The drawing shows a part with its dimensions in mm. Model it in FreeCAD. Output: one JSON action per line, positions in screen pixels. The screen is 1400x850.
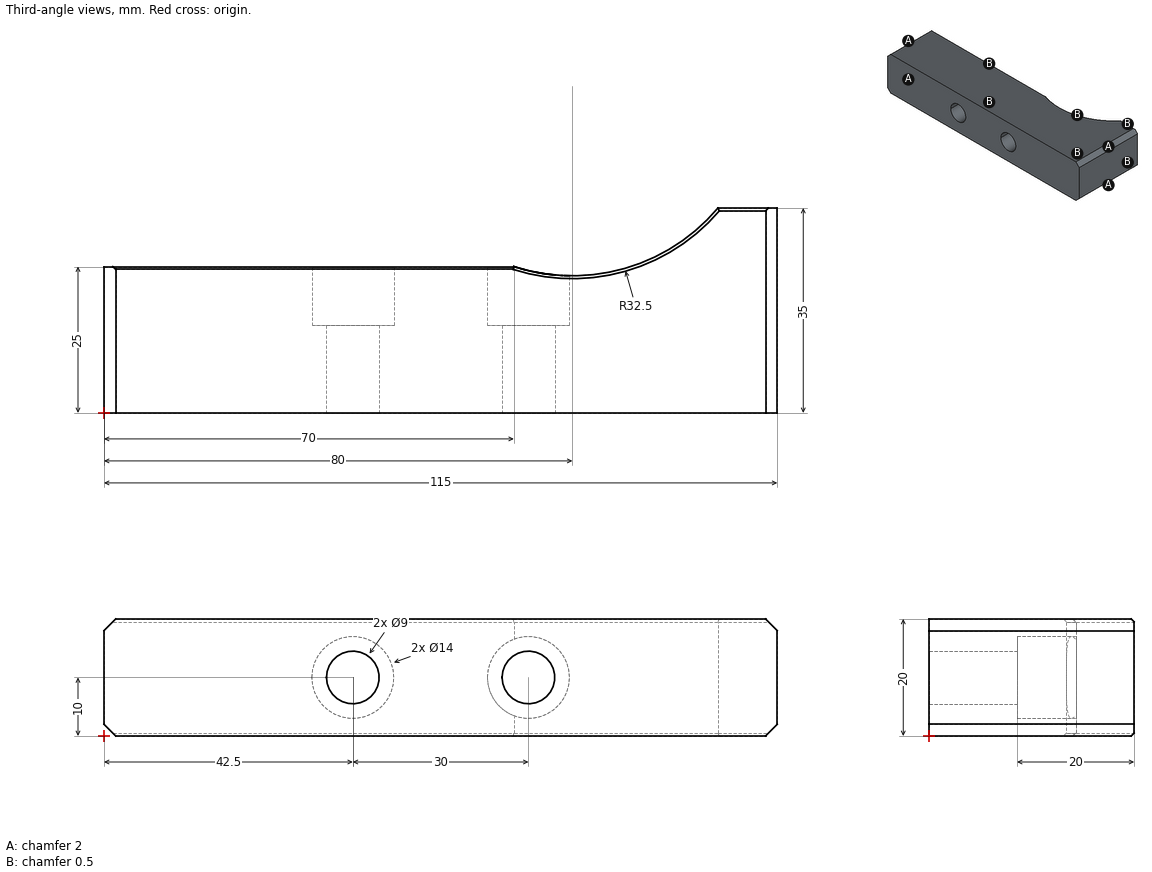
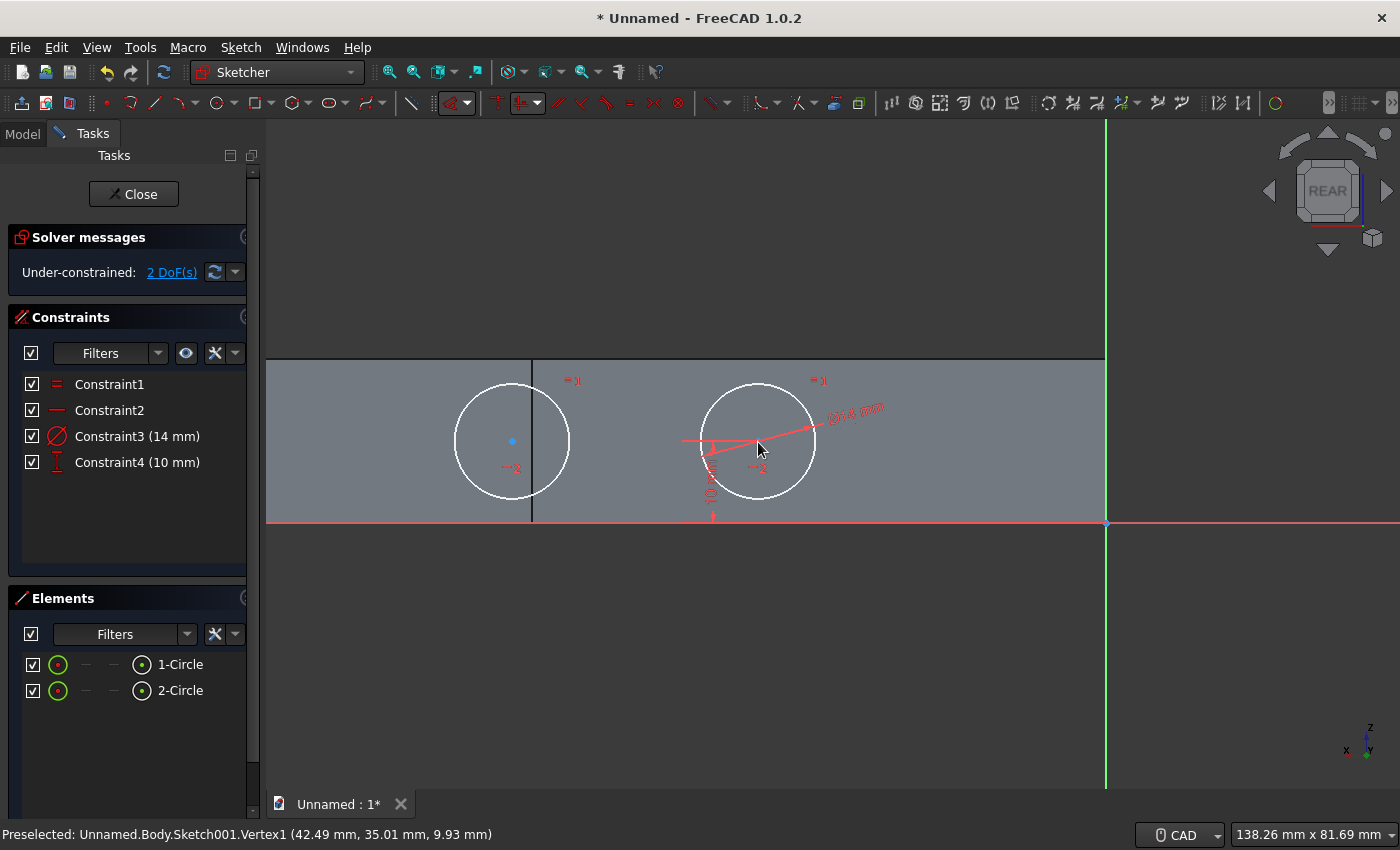
{"action": "left_click", "coordinate": [758, 441]}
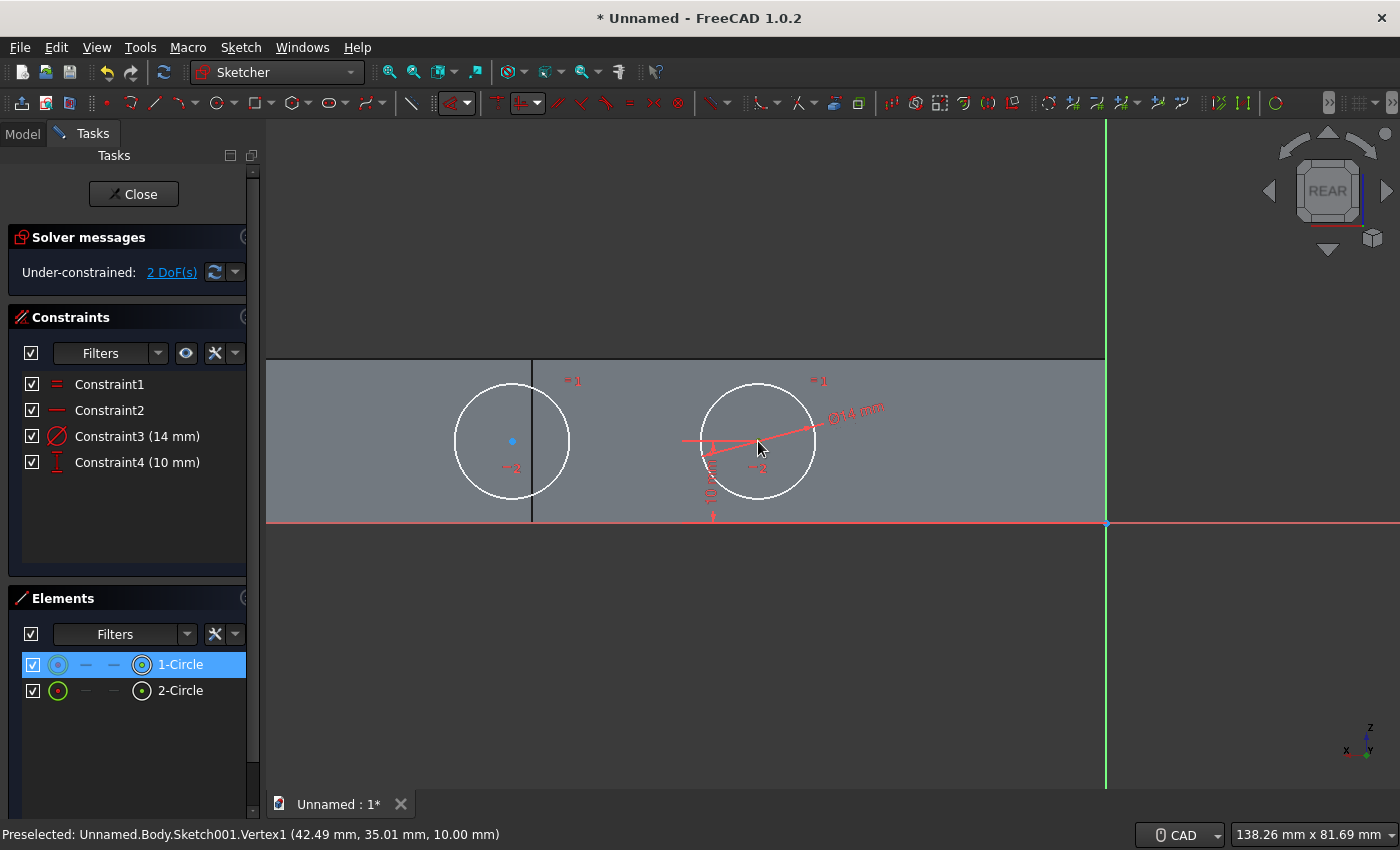
{"action": "left_click", "coordinate": [512, 441]}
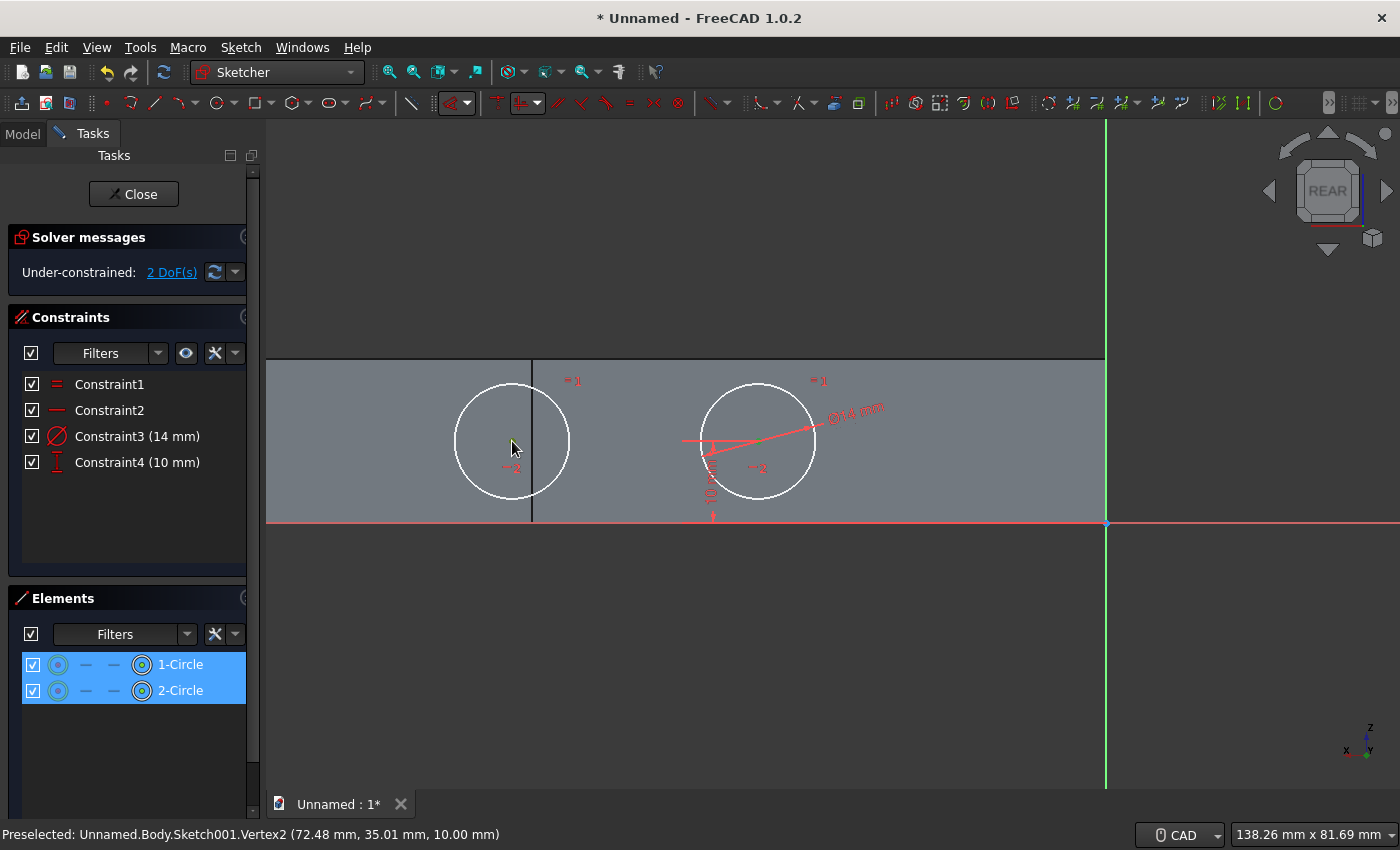
{"action": "left_click", "coordinate": [470, 104]}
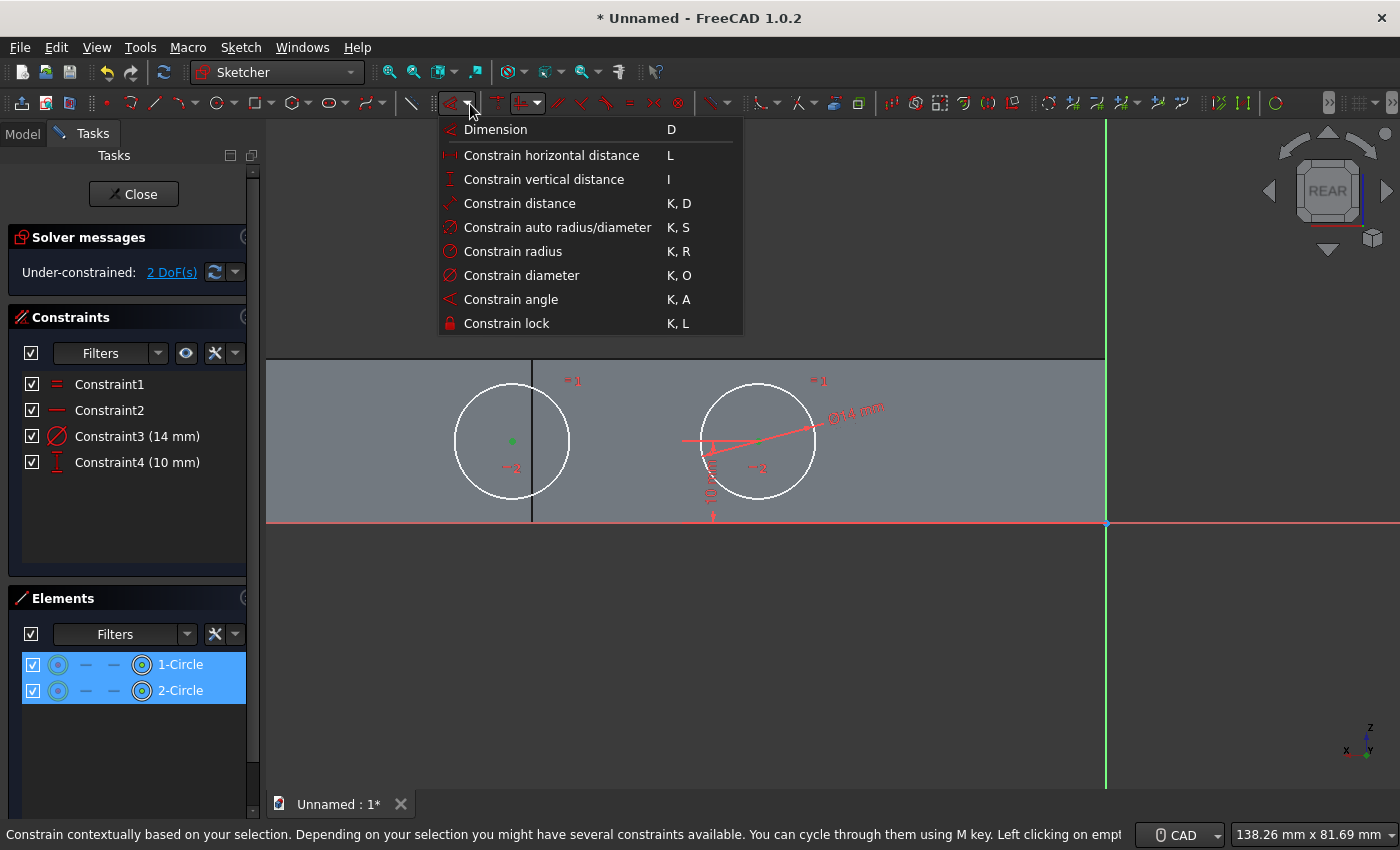
{"action": "left_click", "coordinate": [591, 155]}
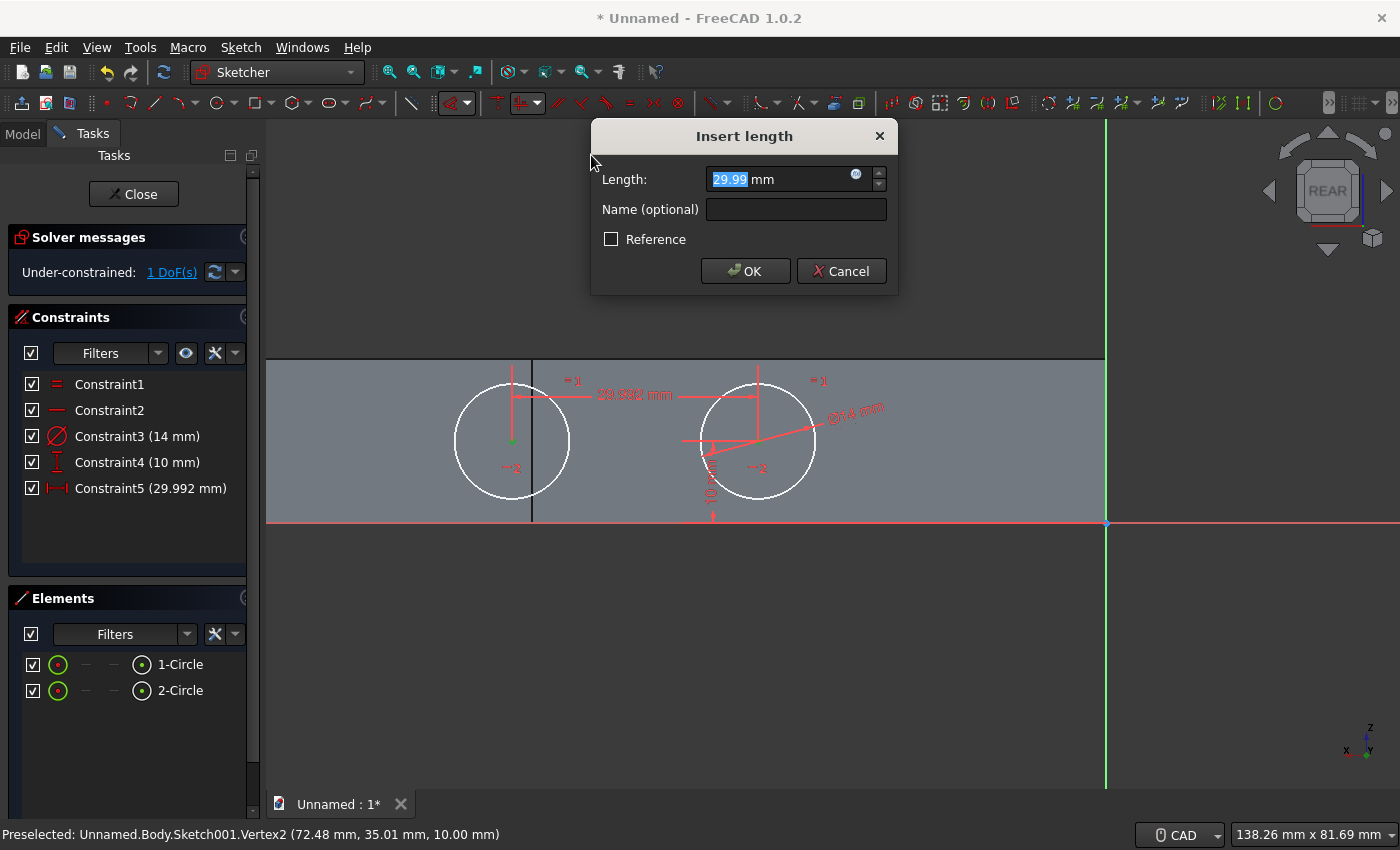
{"action": "type", "text": "30"}
{"action": "key", "text": "Return"}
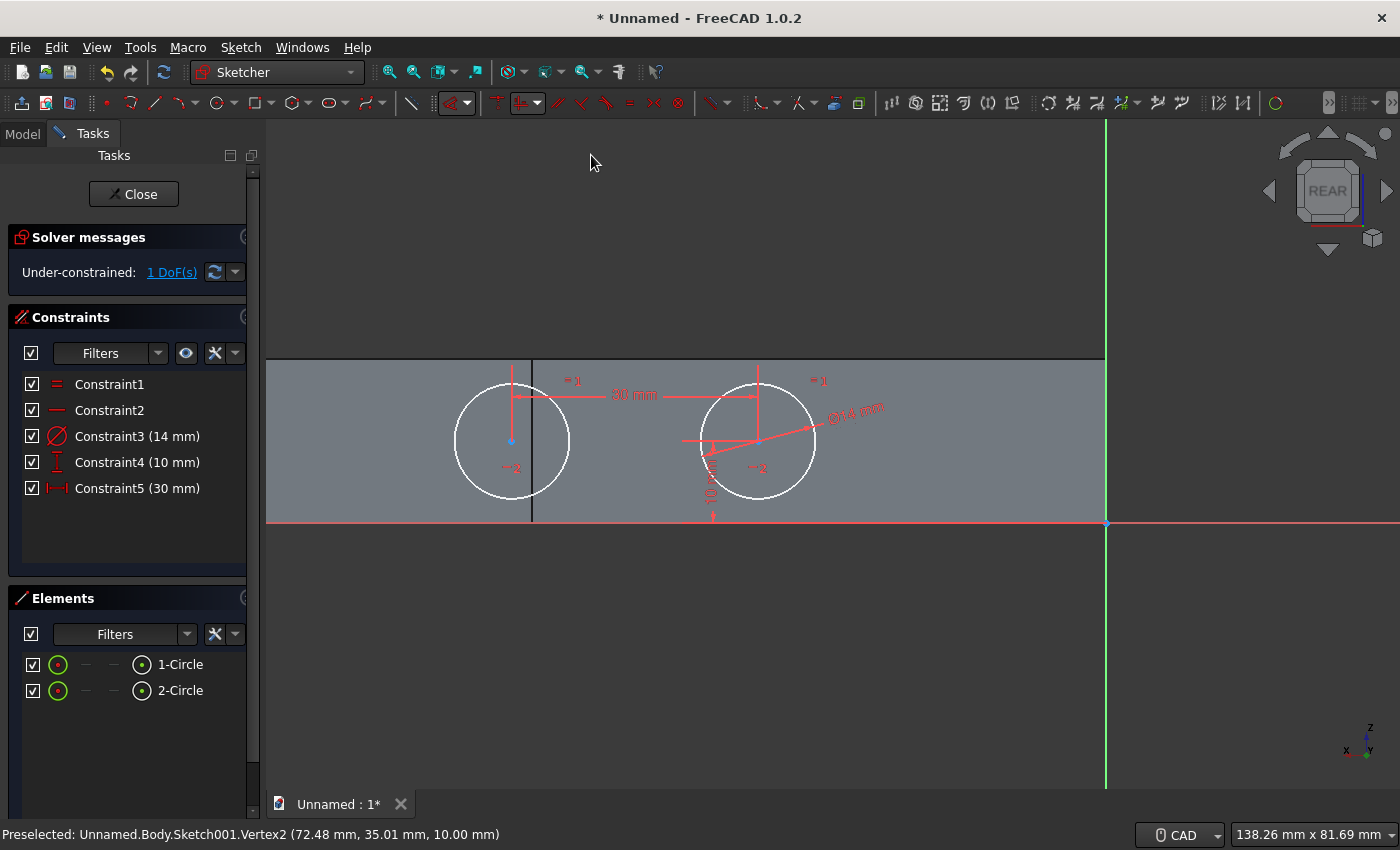
{"action": "left_click", "coordinate": [758, 441]}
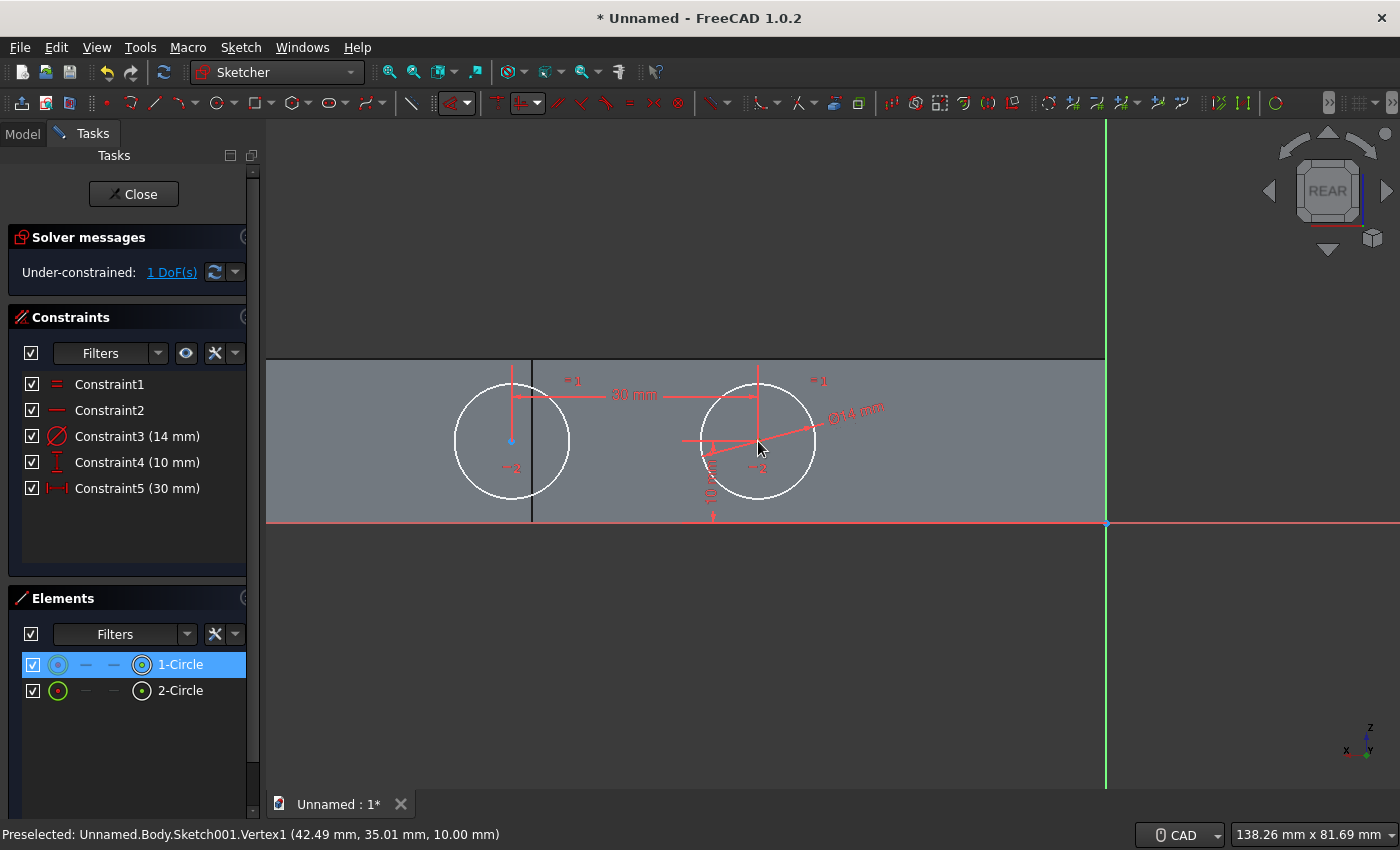
{"action": "key", "text": "l"}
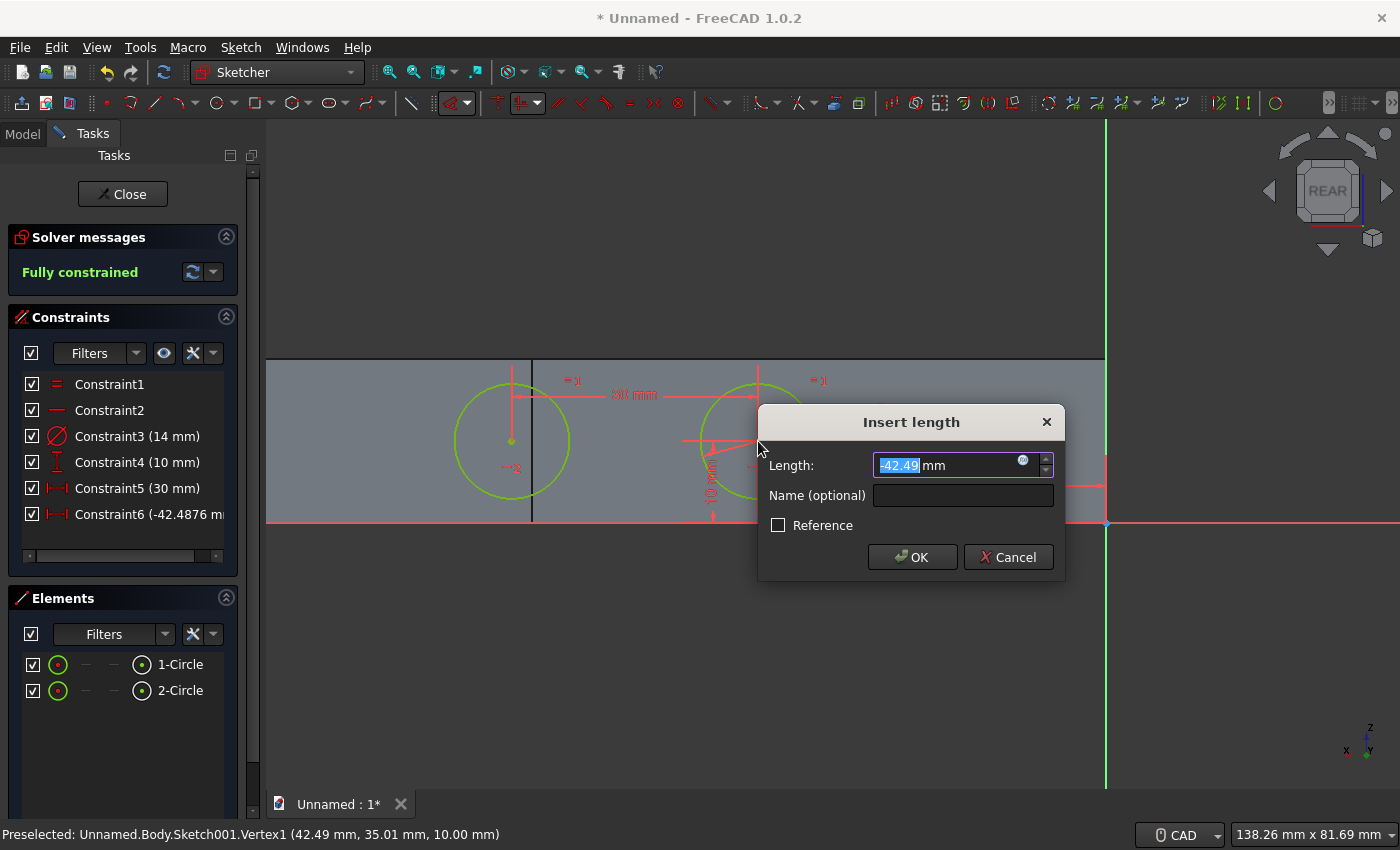
{"action": "type", "text": "-42.5"}
{"action": "key", "text": "Return"}